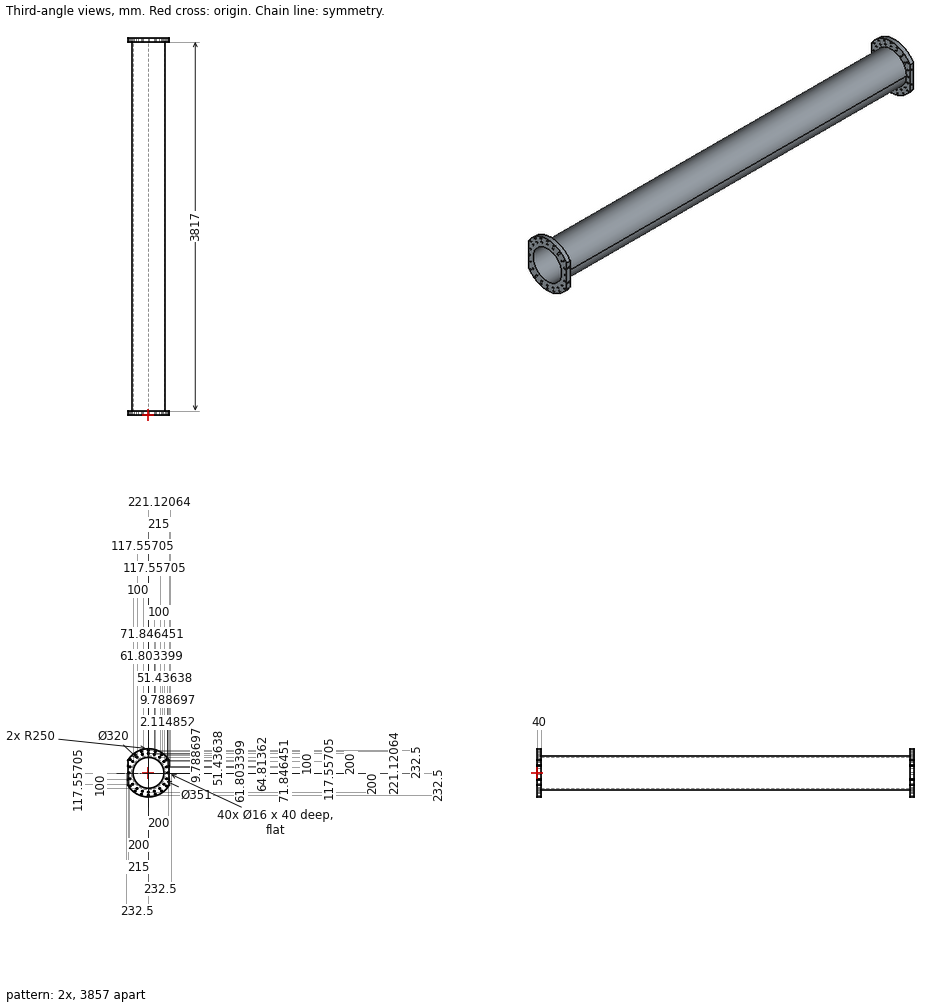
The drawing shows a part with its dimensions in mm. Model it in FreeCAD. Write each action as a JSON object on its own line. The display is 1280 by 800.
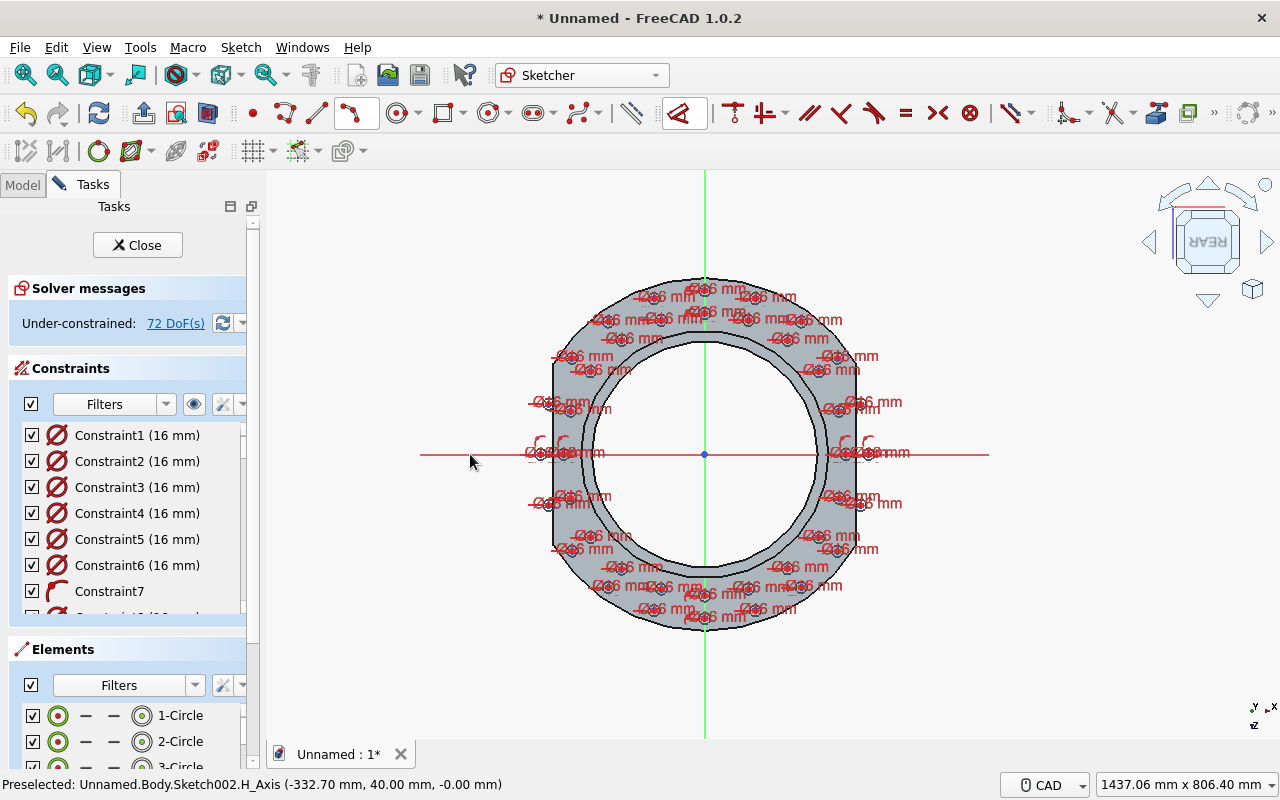
{"action": "left_click", "coordinate": [748, 589]}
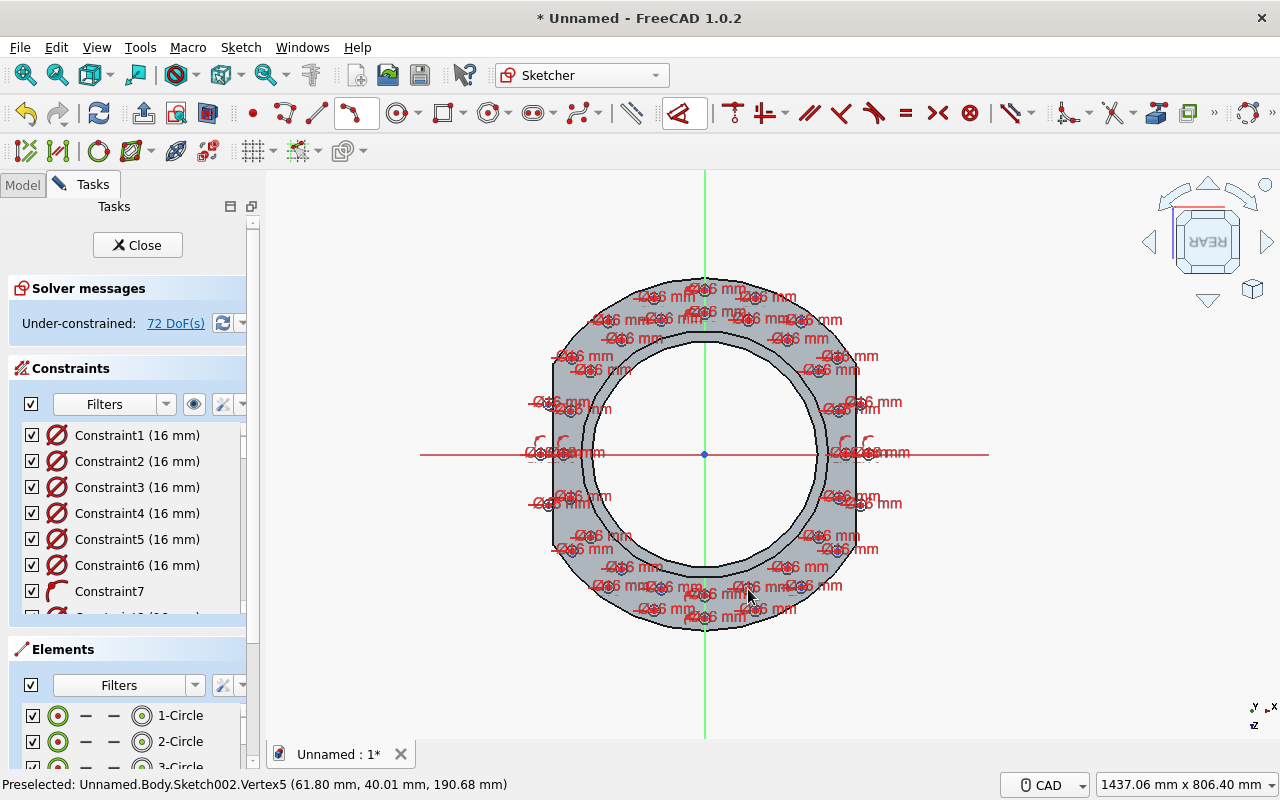
{"action": "left_click", "coordinate": [661, 589]}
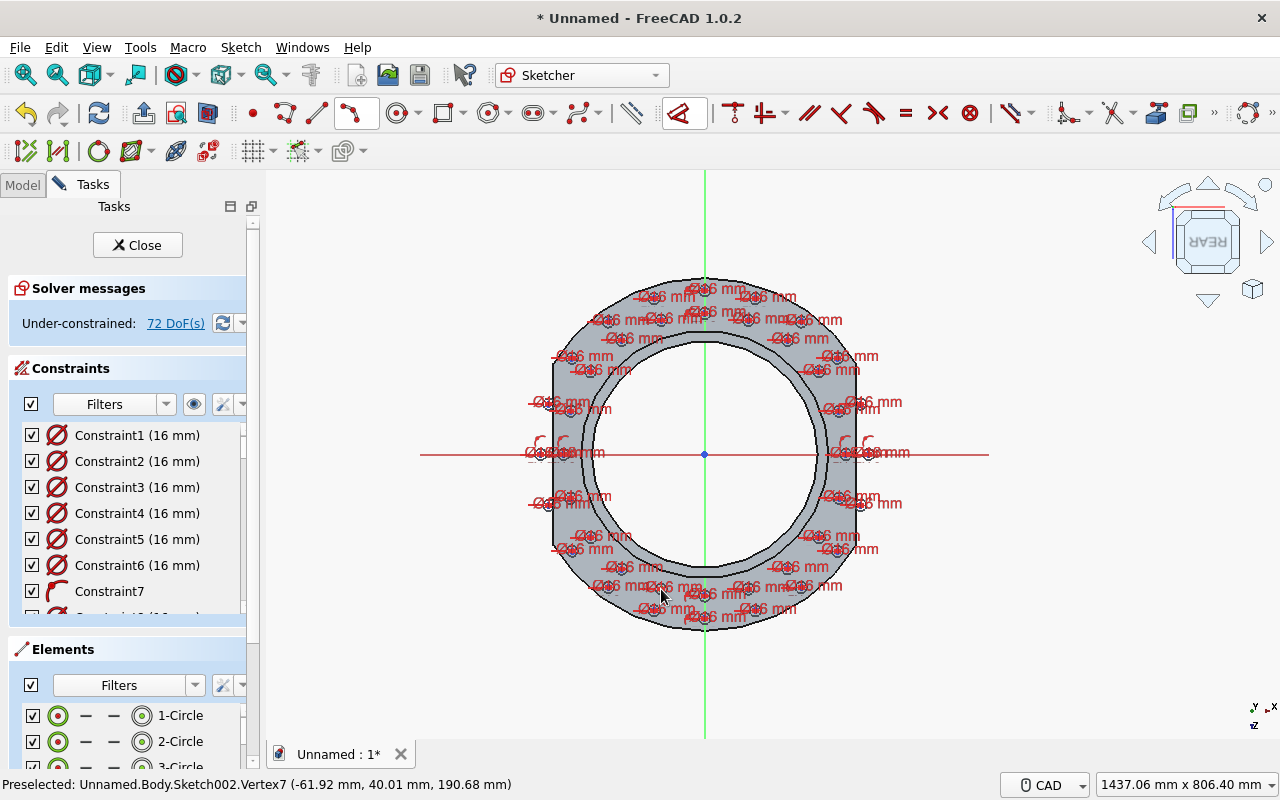
{"action": "key", "text": "h"}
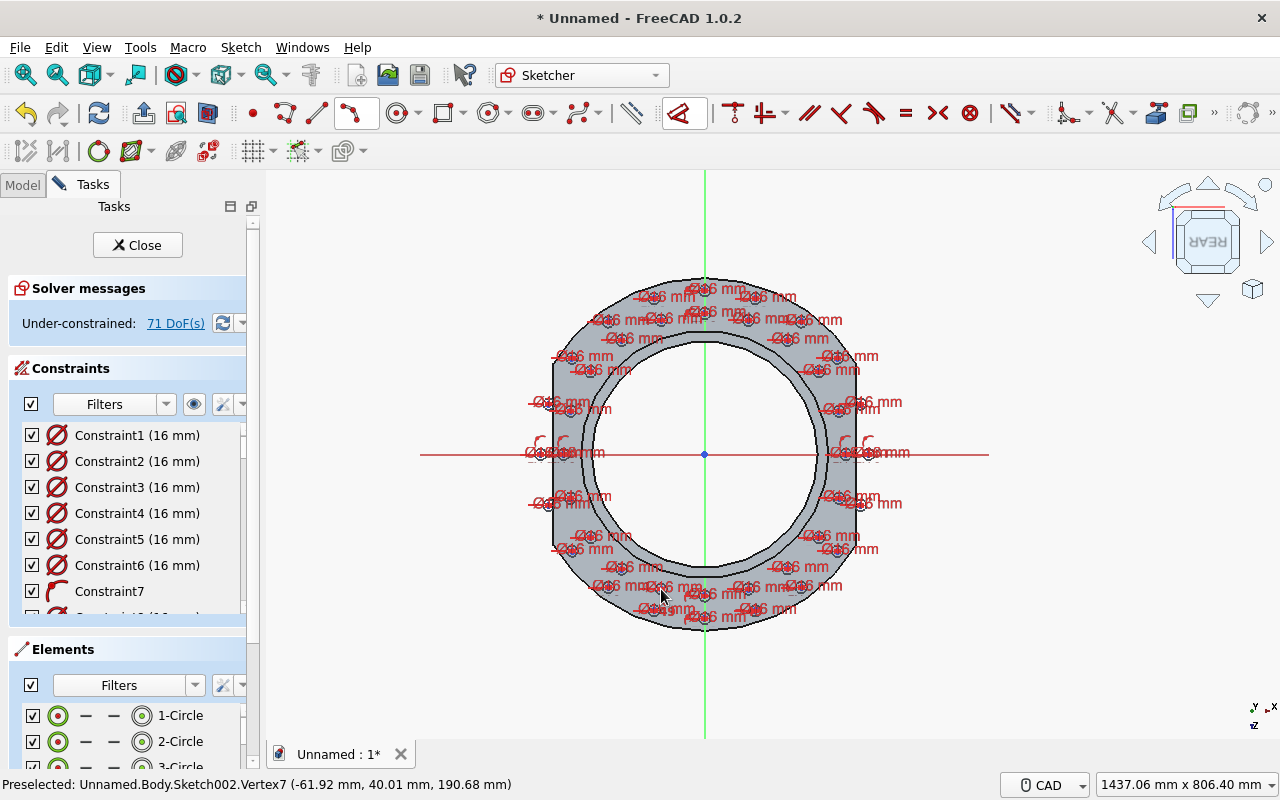
{"action": "left_click", "coordinate": [788, 569]}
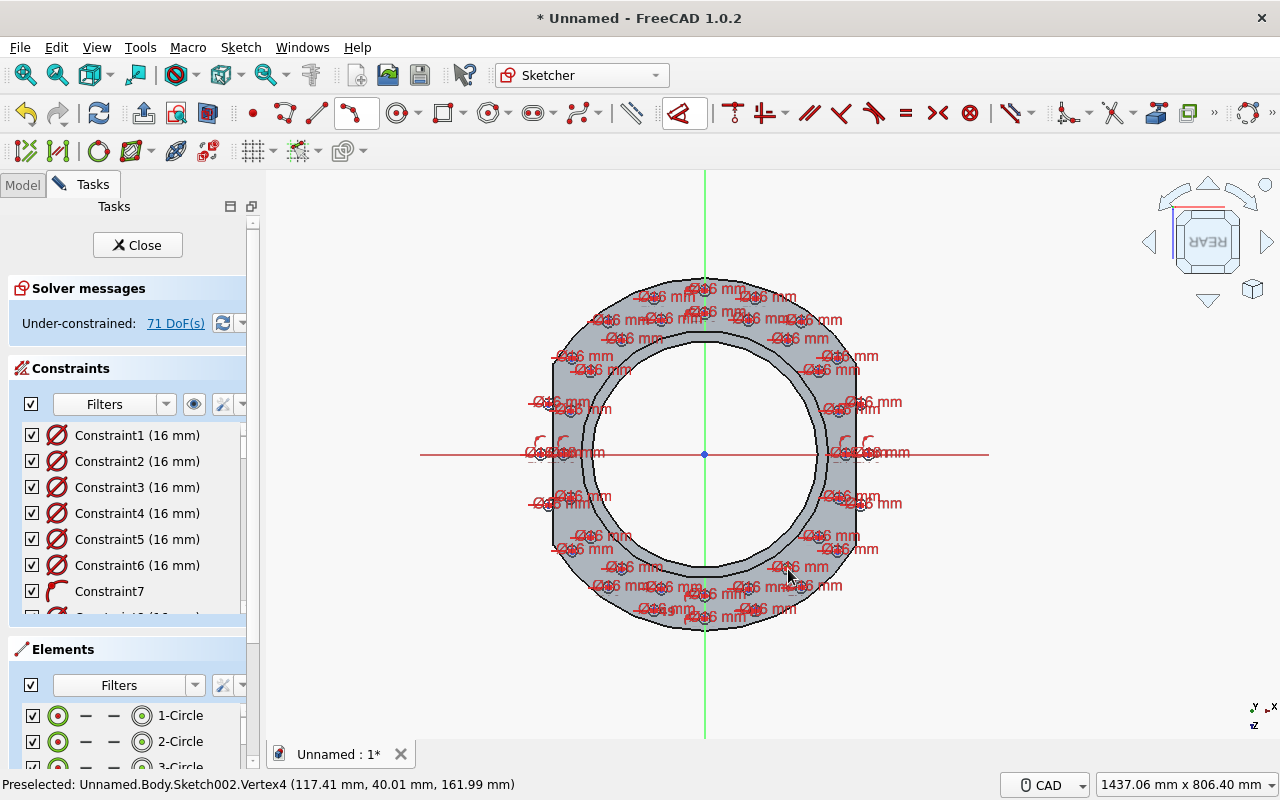
{"action": "left_click", "coordinate": [622, 569]}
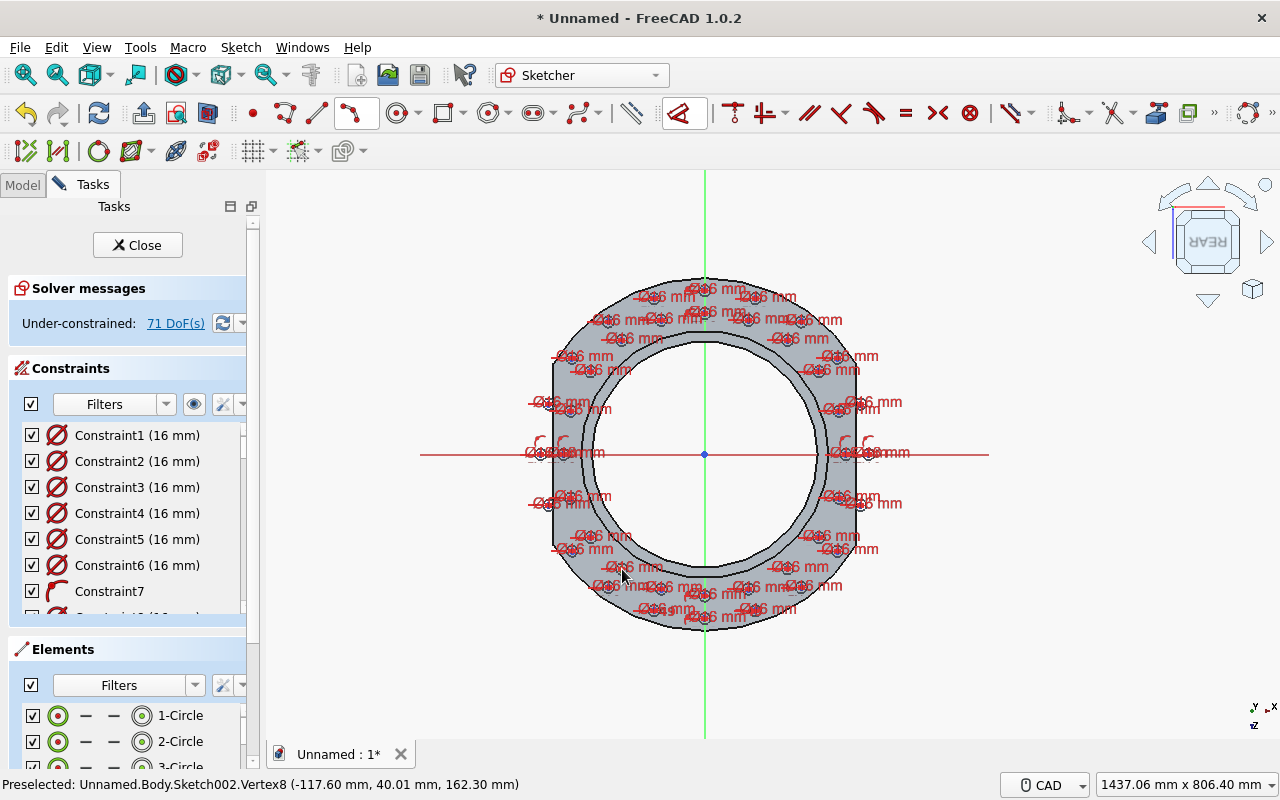
{"action": "left_click", "coordinate": [788, 114]}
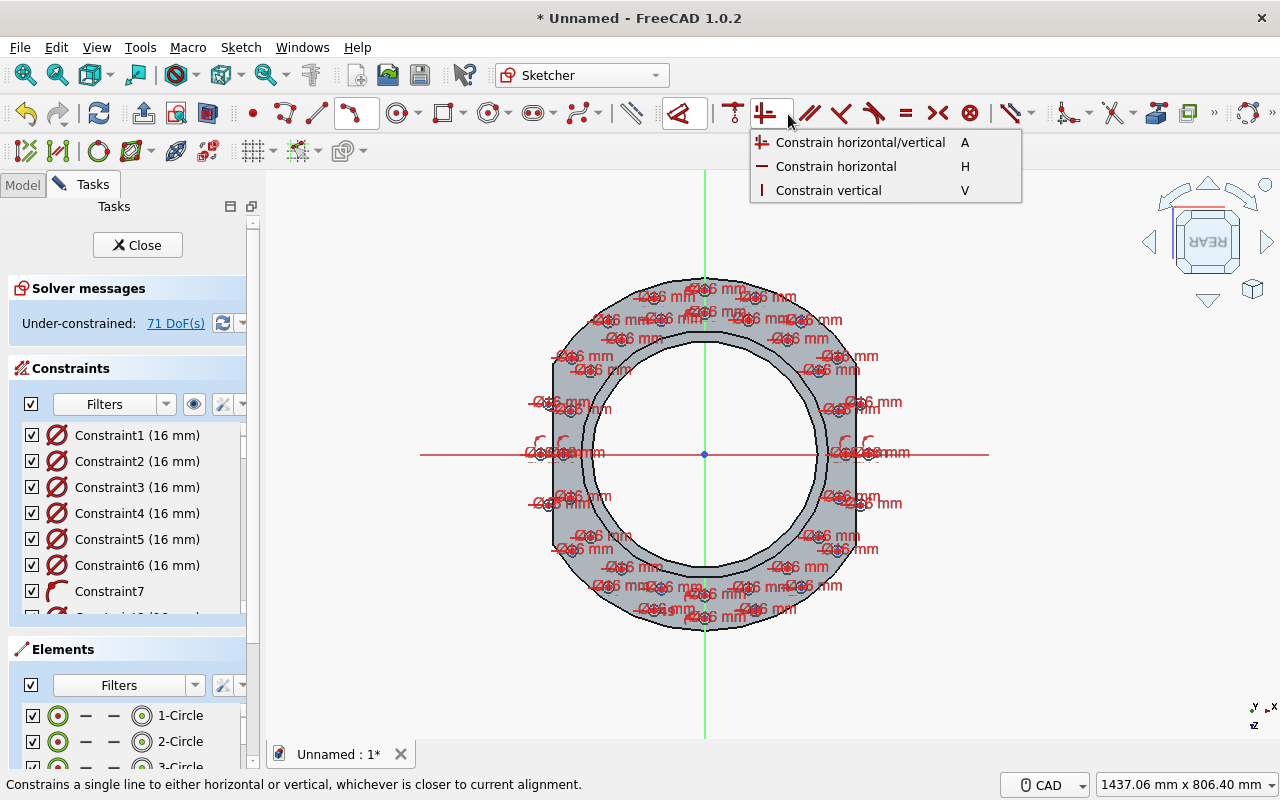
{"action": "left_click", "coordinate": [886, 166]}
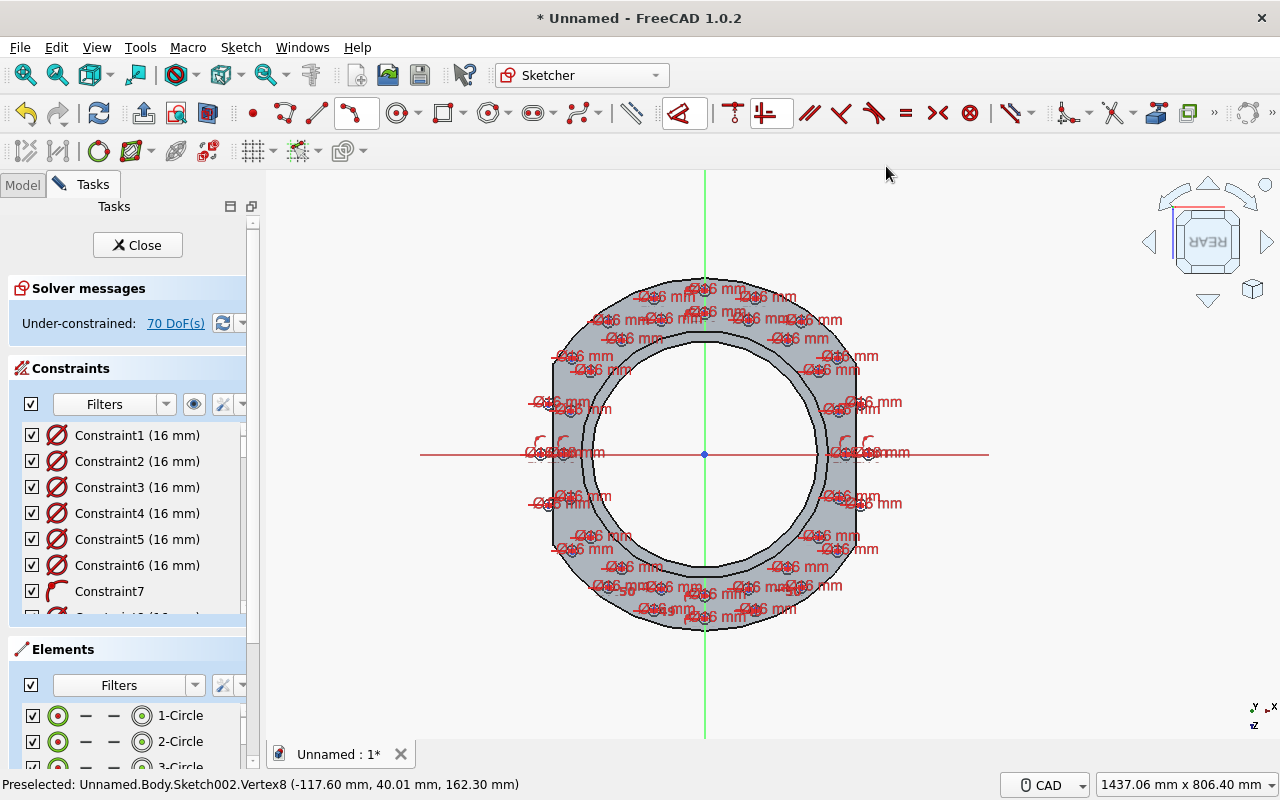
{"action": "left_click", "coordinate": [819, 538]}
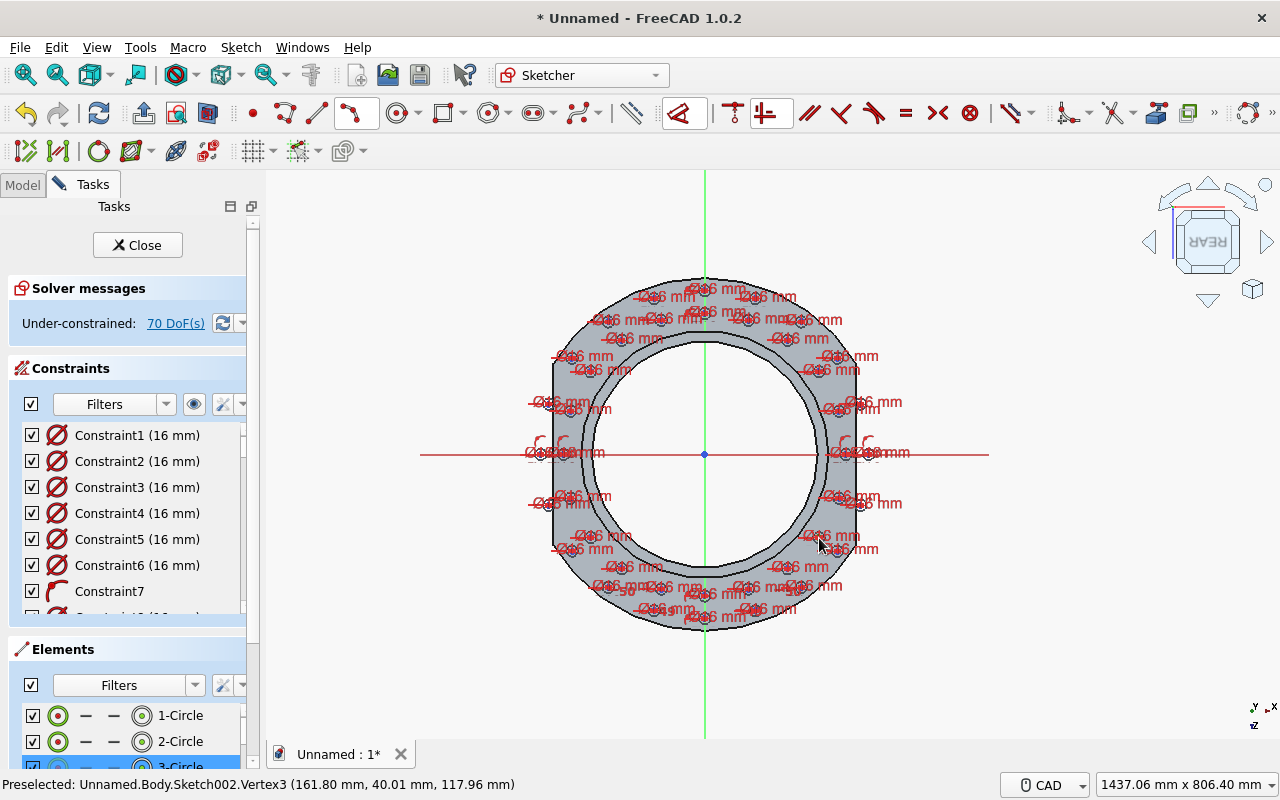
{"action": "left_click", "coordinate": [591, 538]}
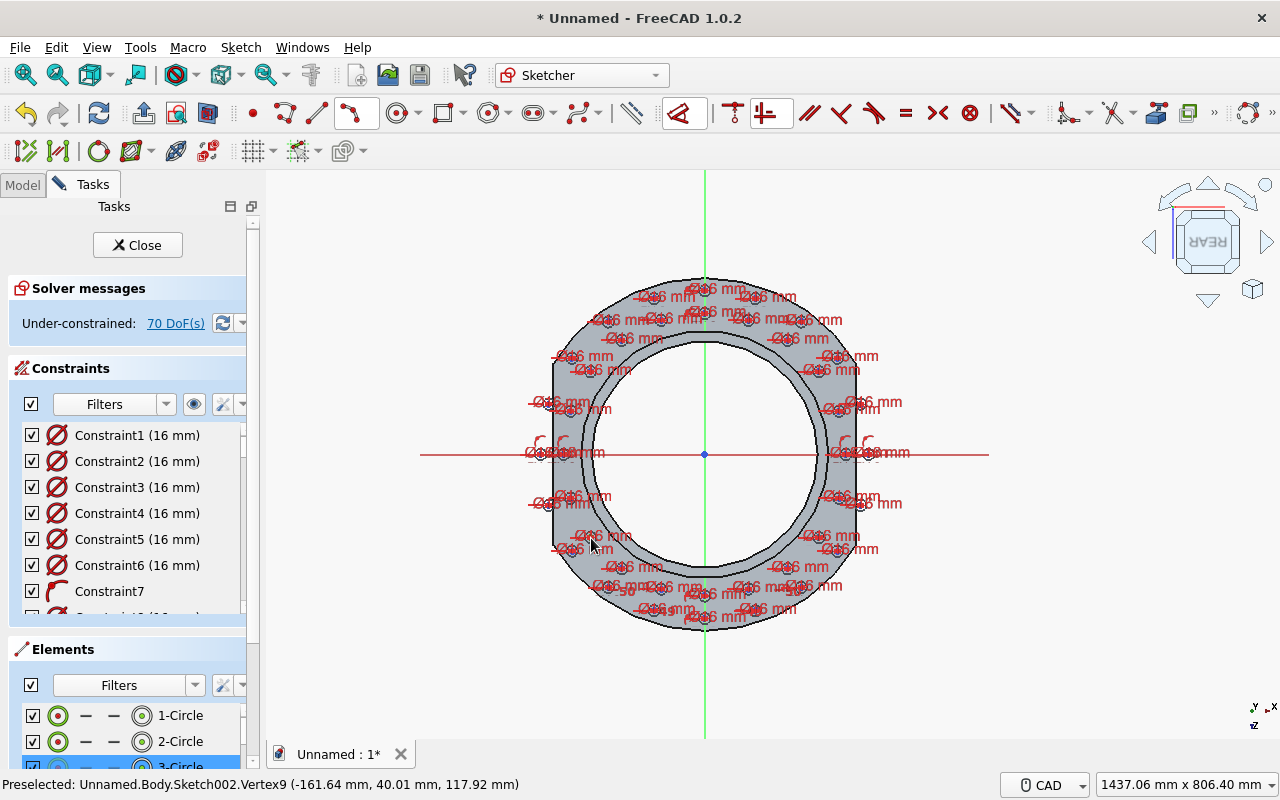
{"action": "left_click", "coordinate": [788, 114]}